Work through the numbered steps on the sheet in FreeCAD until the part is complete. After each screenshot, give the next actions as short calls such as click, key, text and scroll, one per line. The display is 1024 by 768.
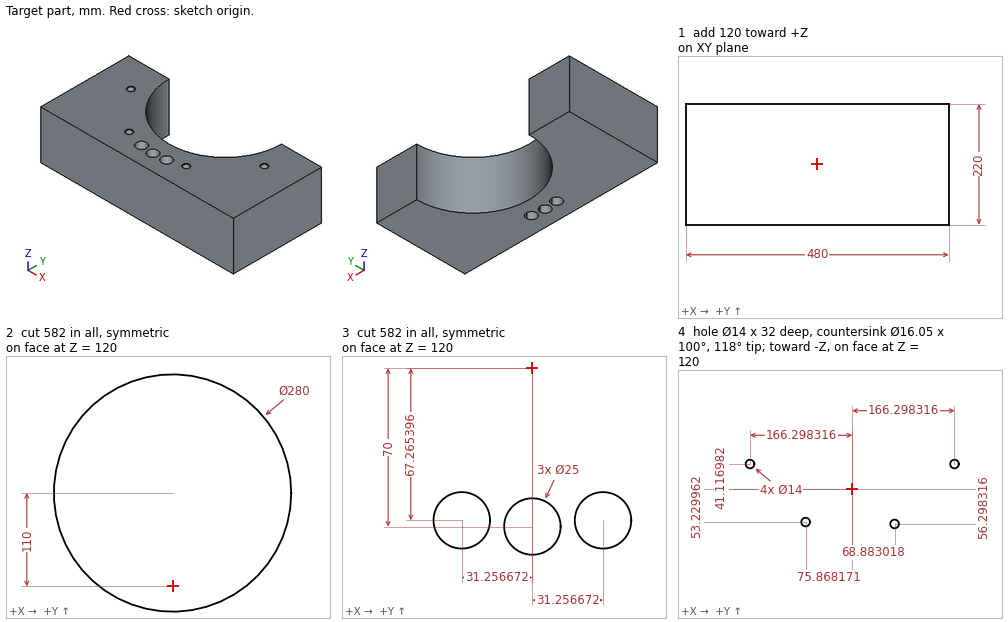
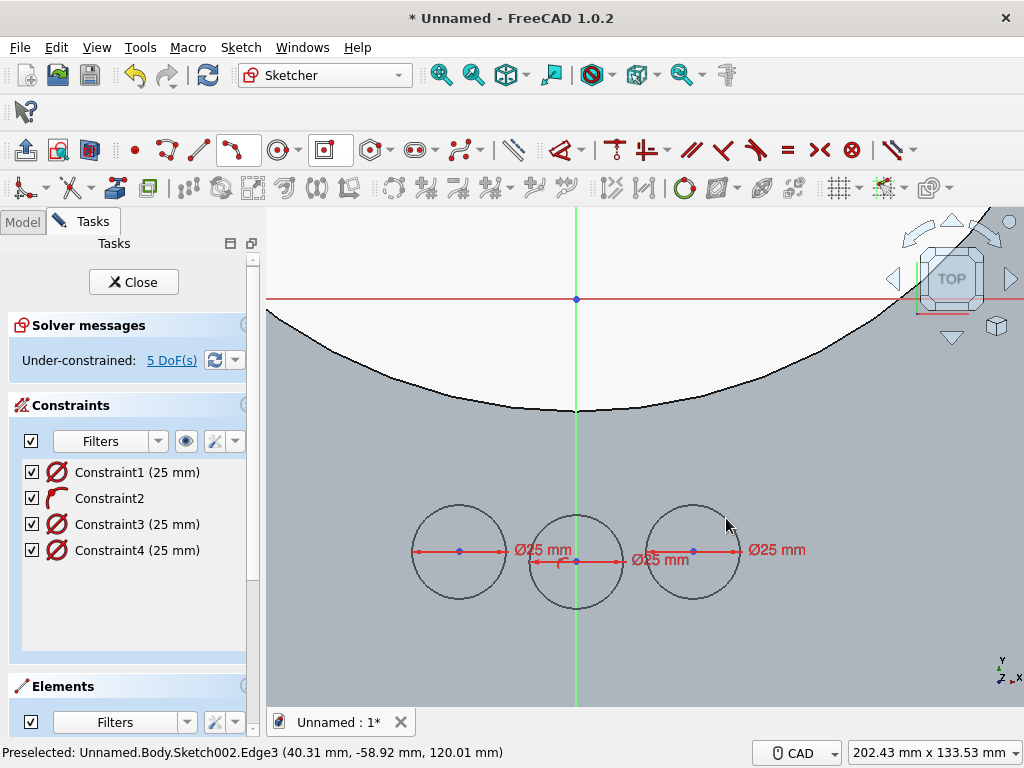
click(459, 552)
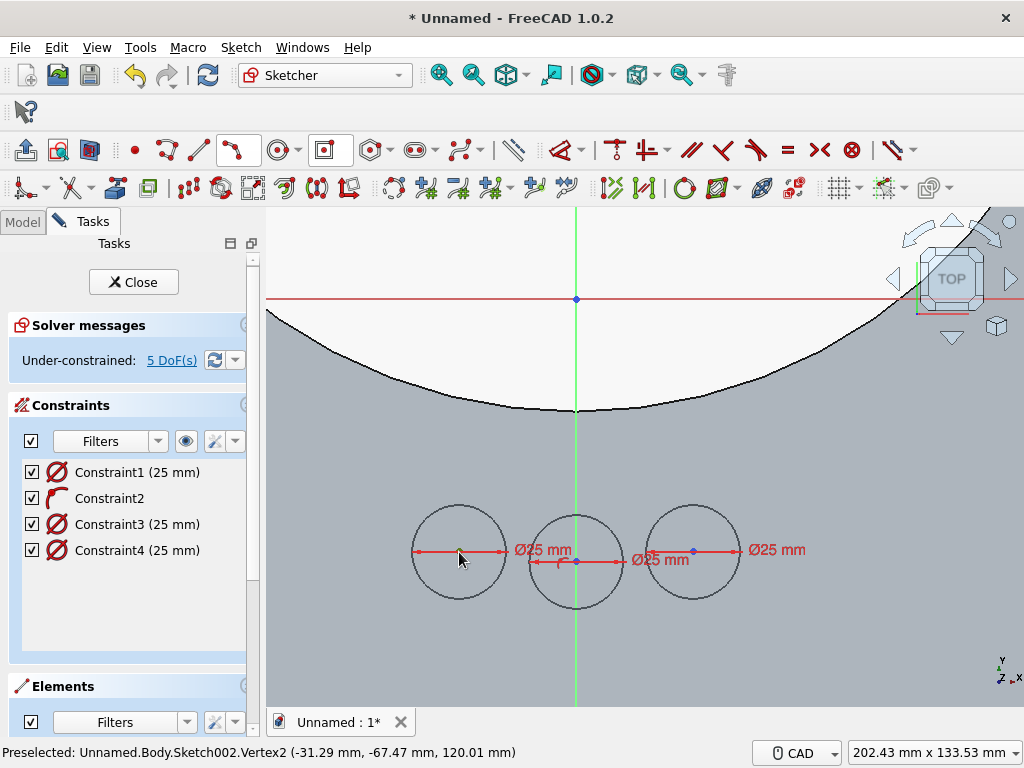
click(693, 552)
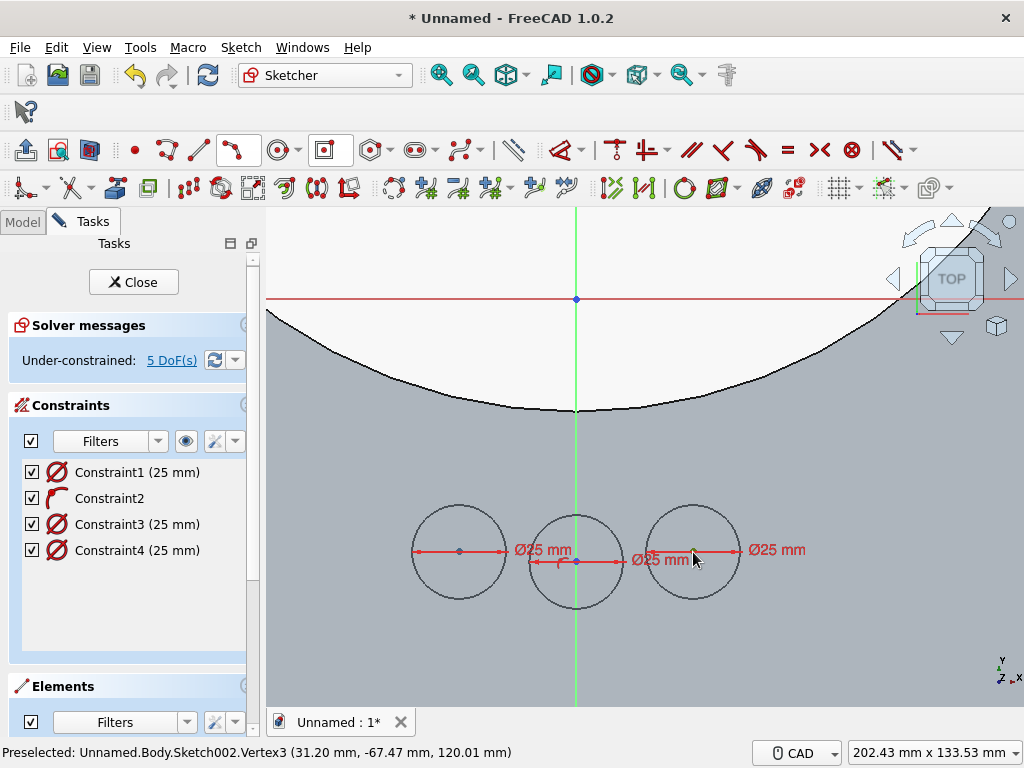
key(h)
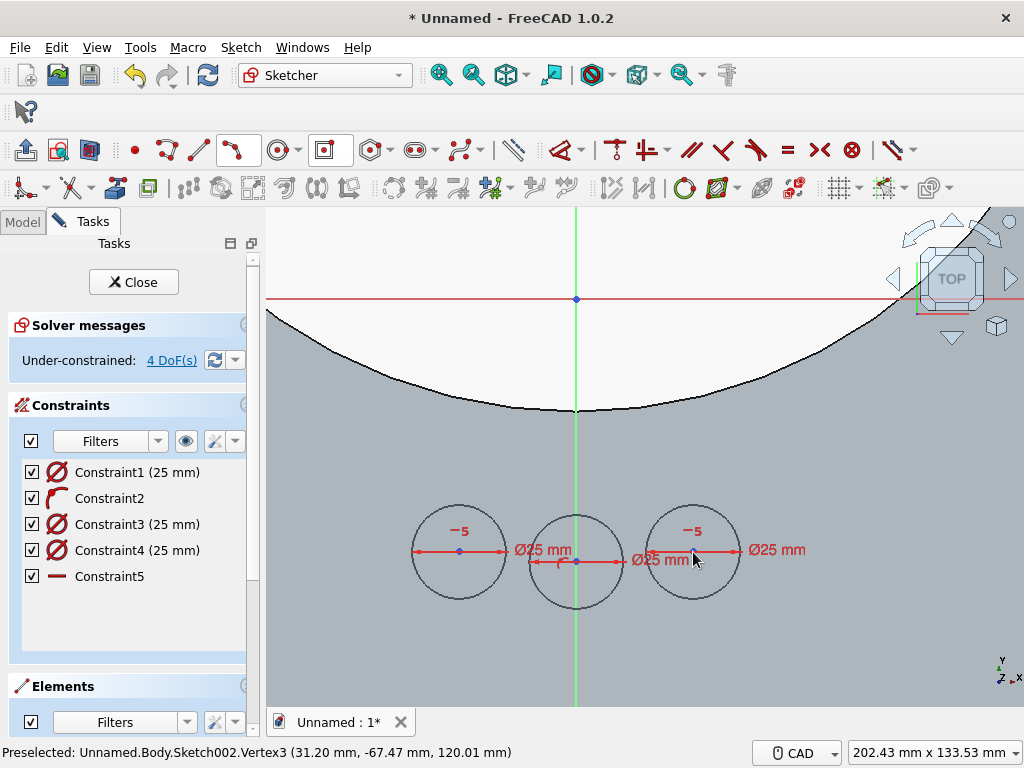
key(d)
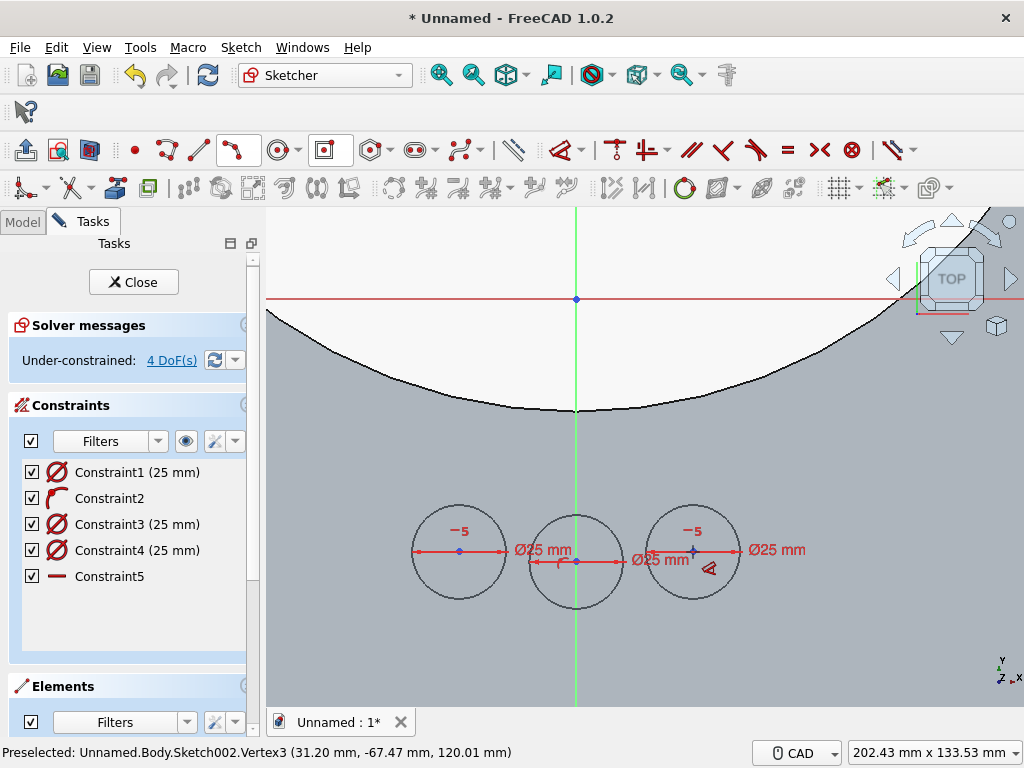
click(576, 562)
click(610, 431)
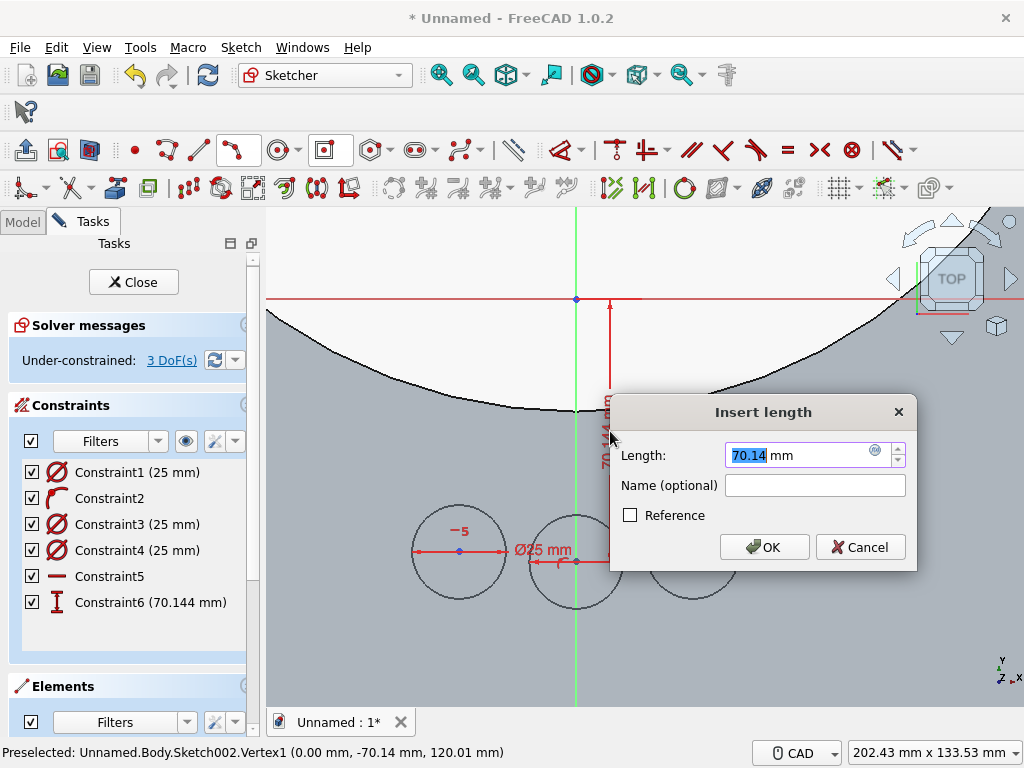
text(70)
key(Return)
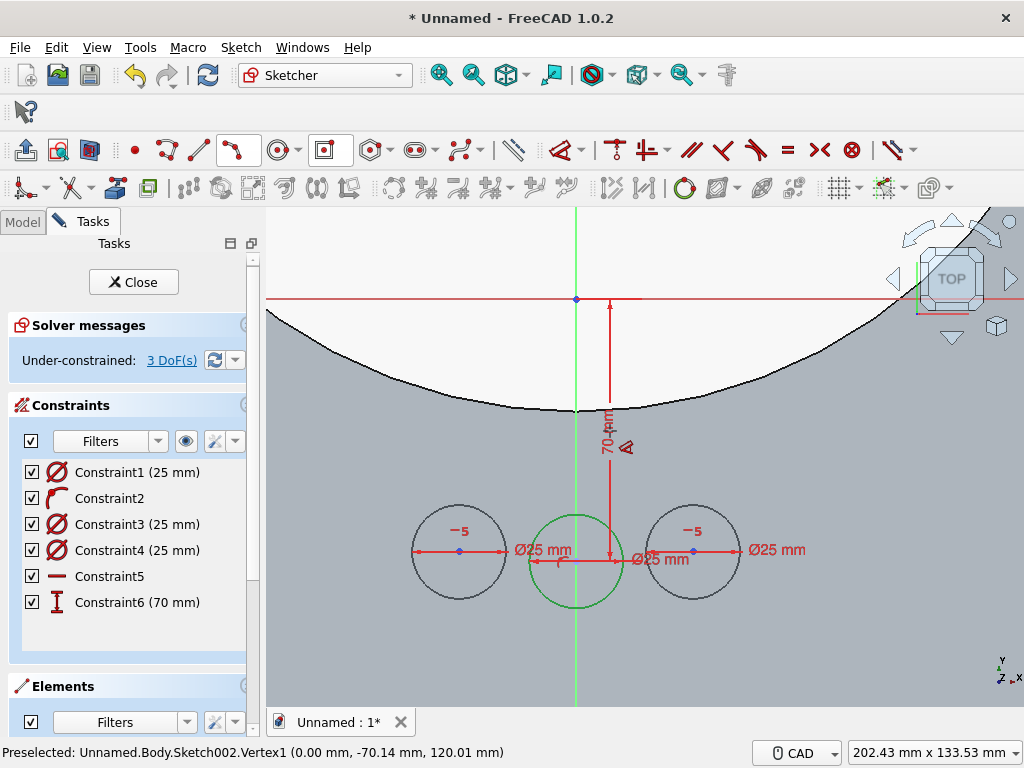
click(459, 552)
click(518, 265)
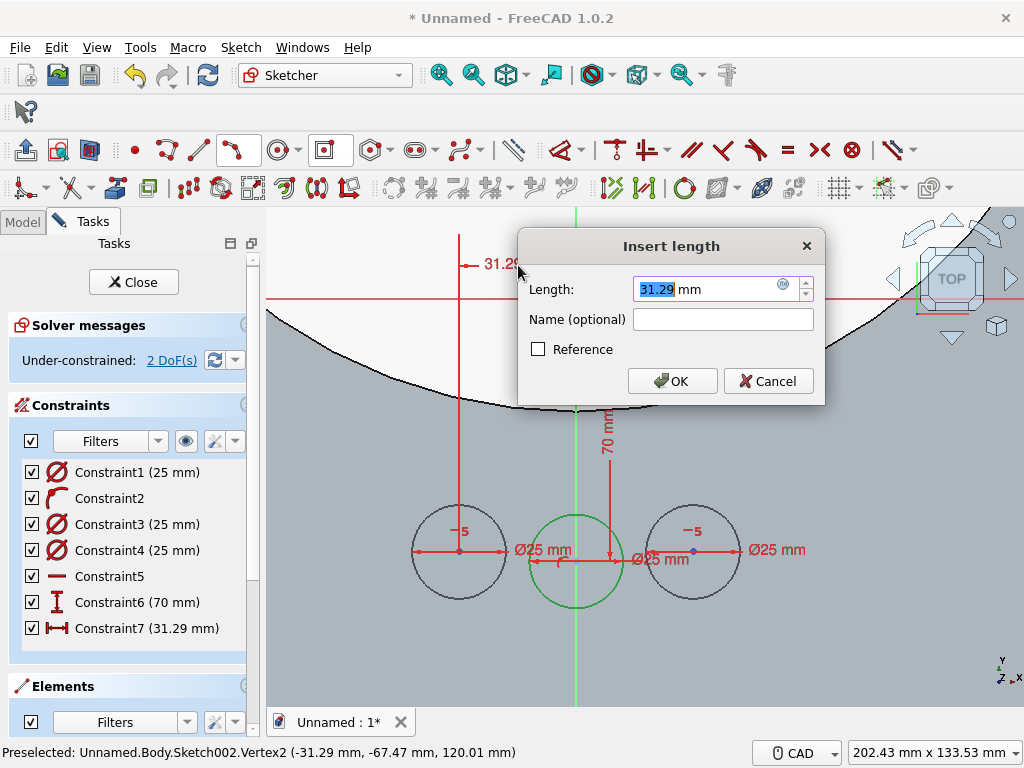
text(31.256672)
key(Return)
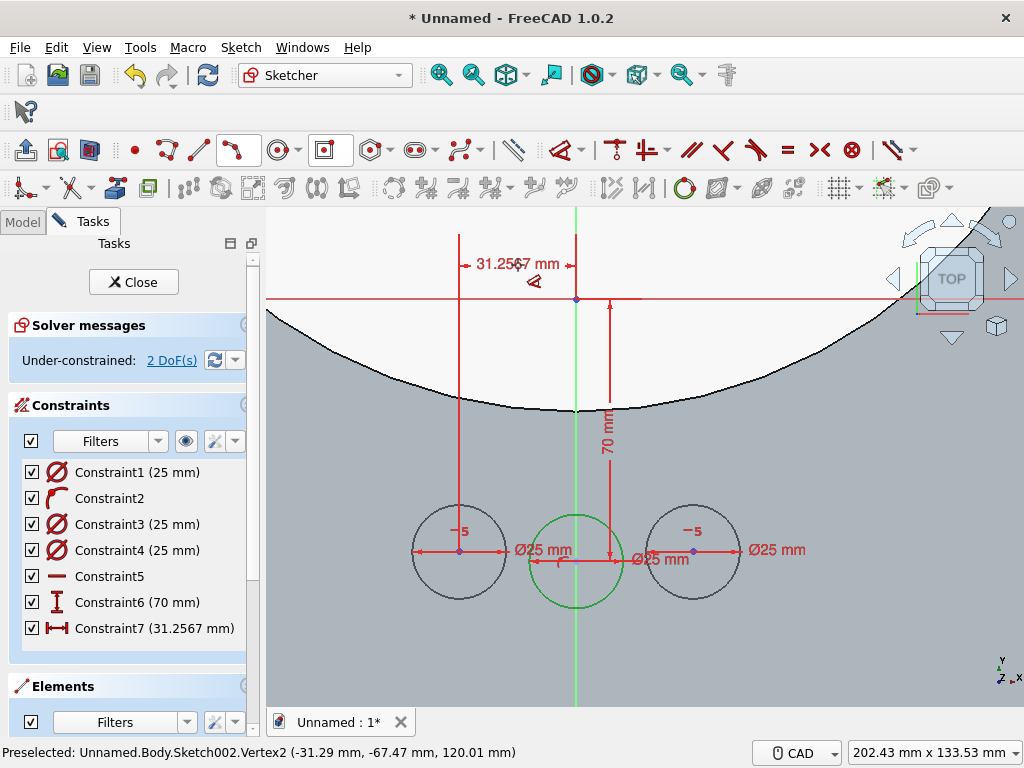
click(459, 552)
click(425, 426)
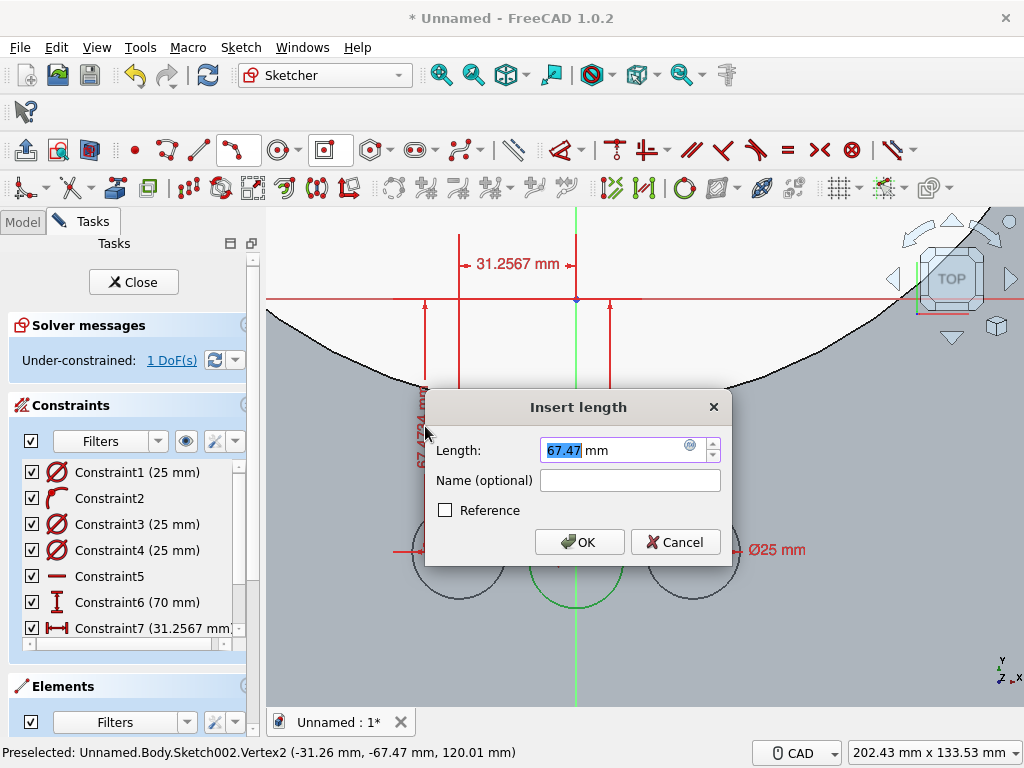
text(67.265396)
key(Return)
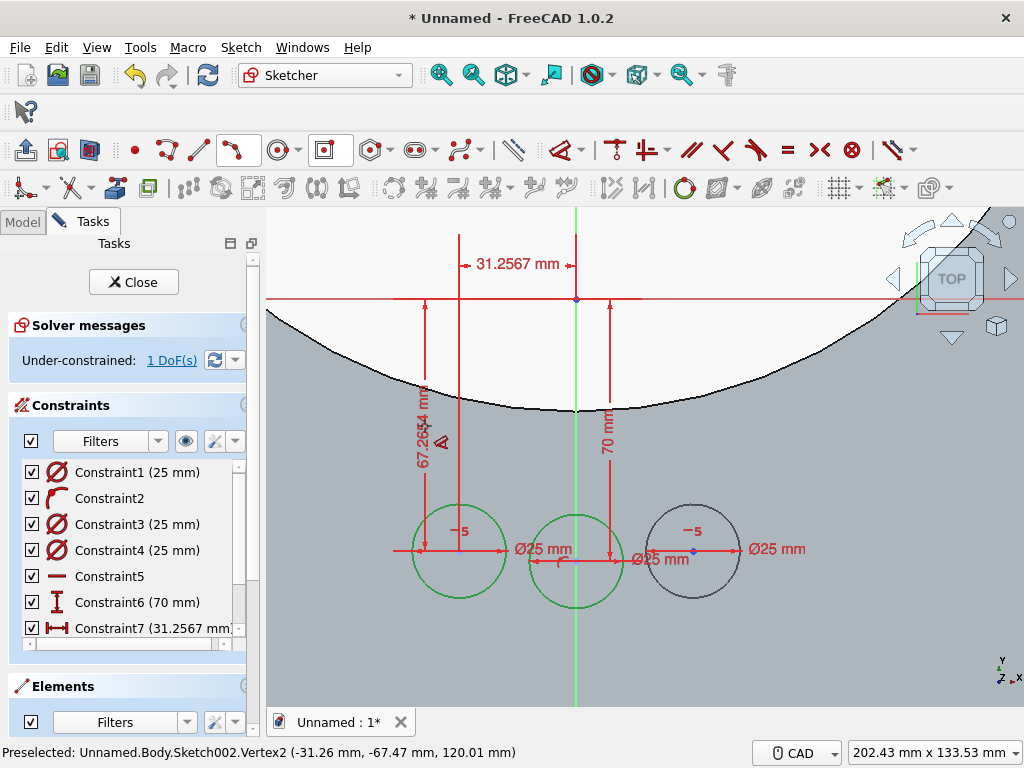
click(693, 551)
click(635, 265)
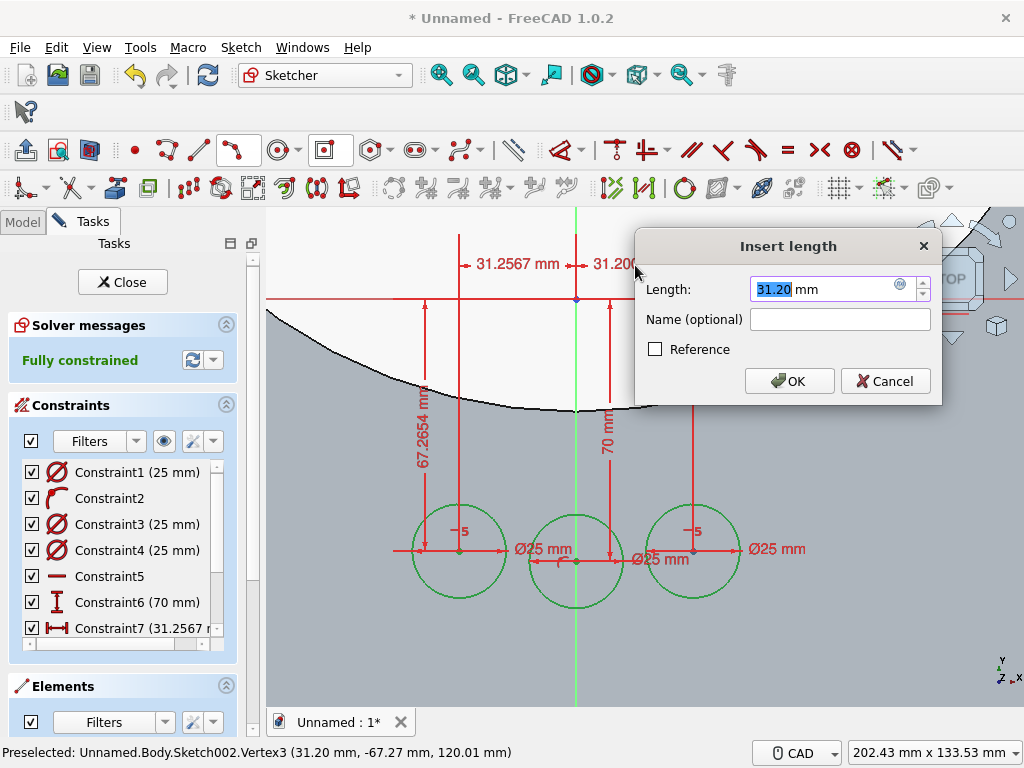
text(31.256672)
key(Return)
key(Escape)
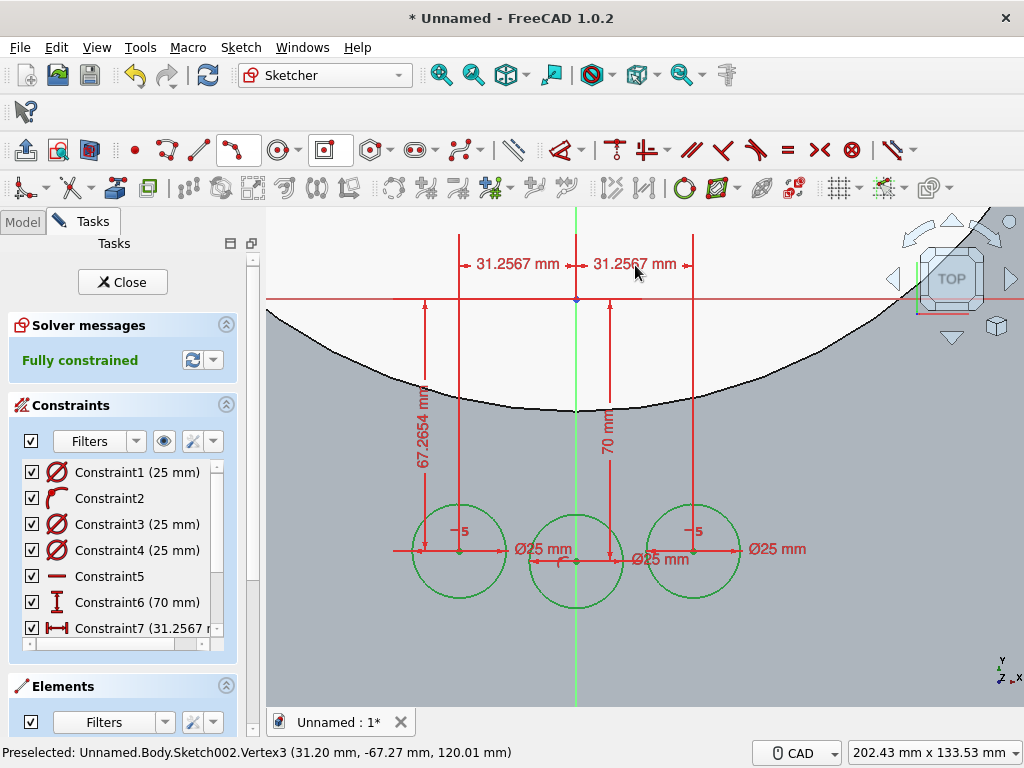
click(123, 282)